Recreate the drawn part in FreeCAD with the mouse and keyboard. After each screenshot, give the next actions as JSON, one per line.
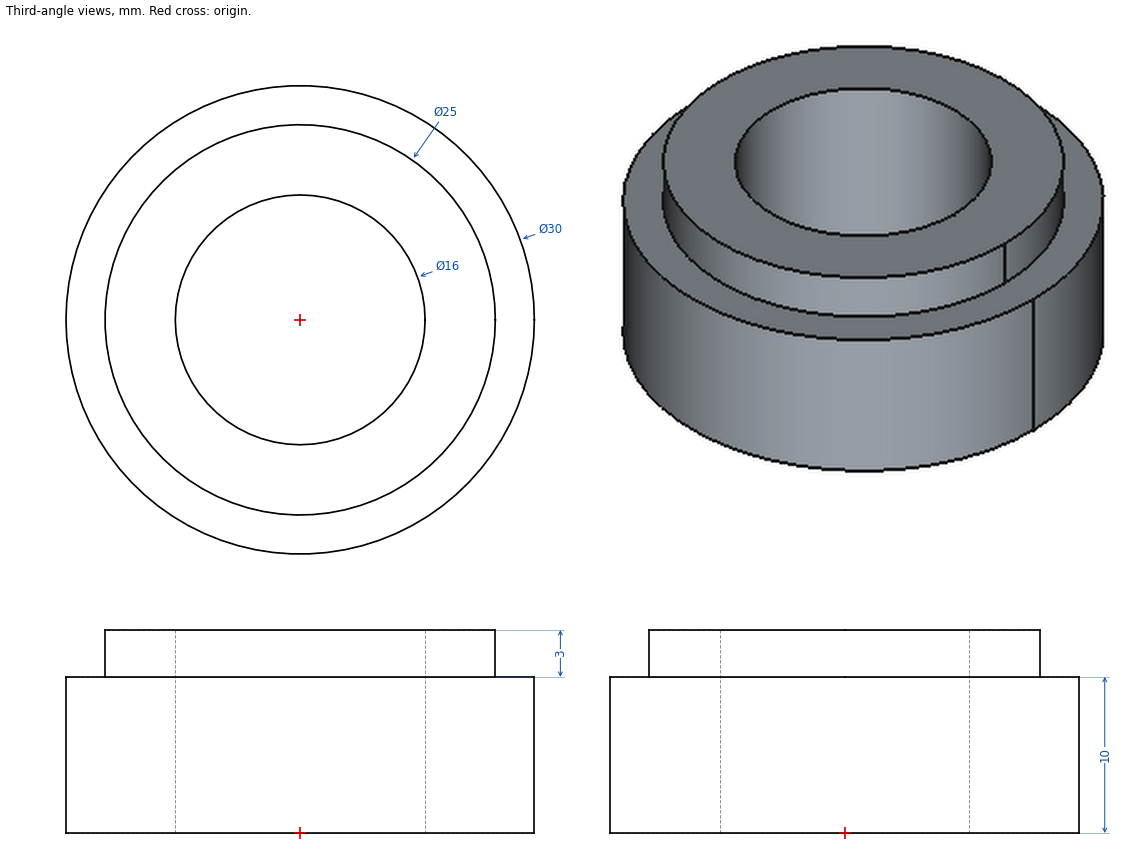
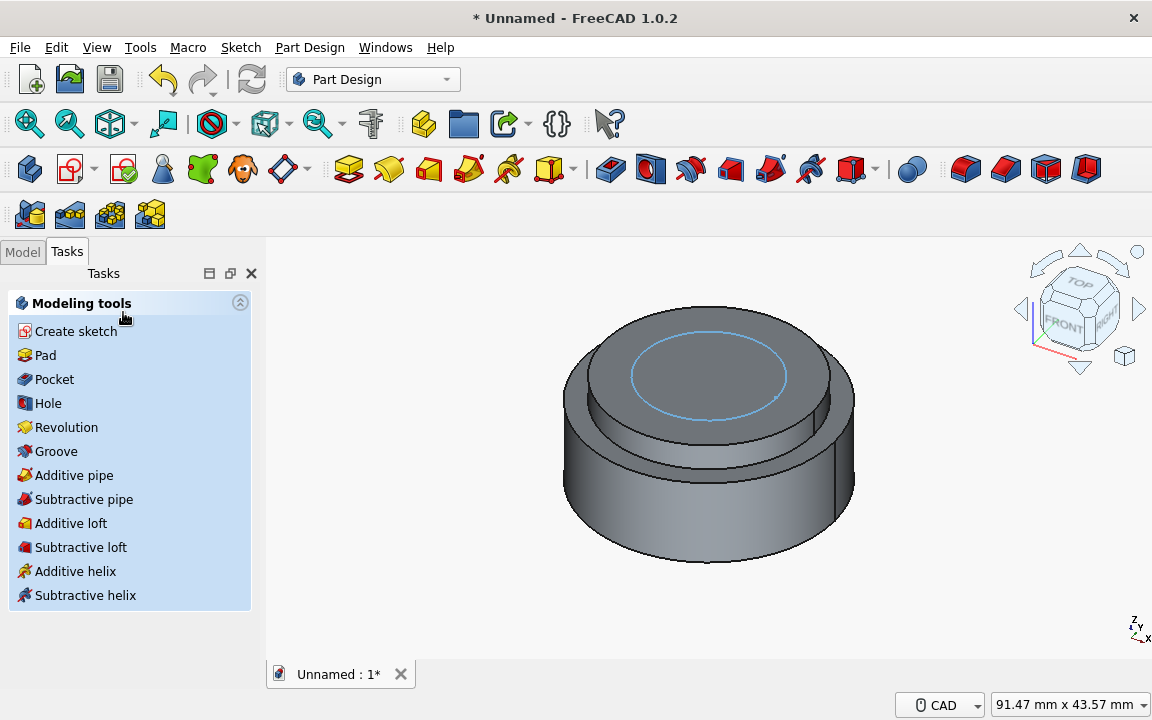
{"action": "left_click", "coordinate": [612, 170]}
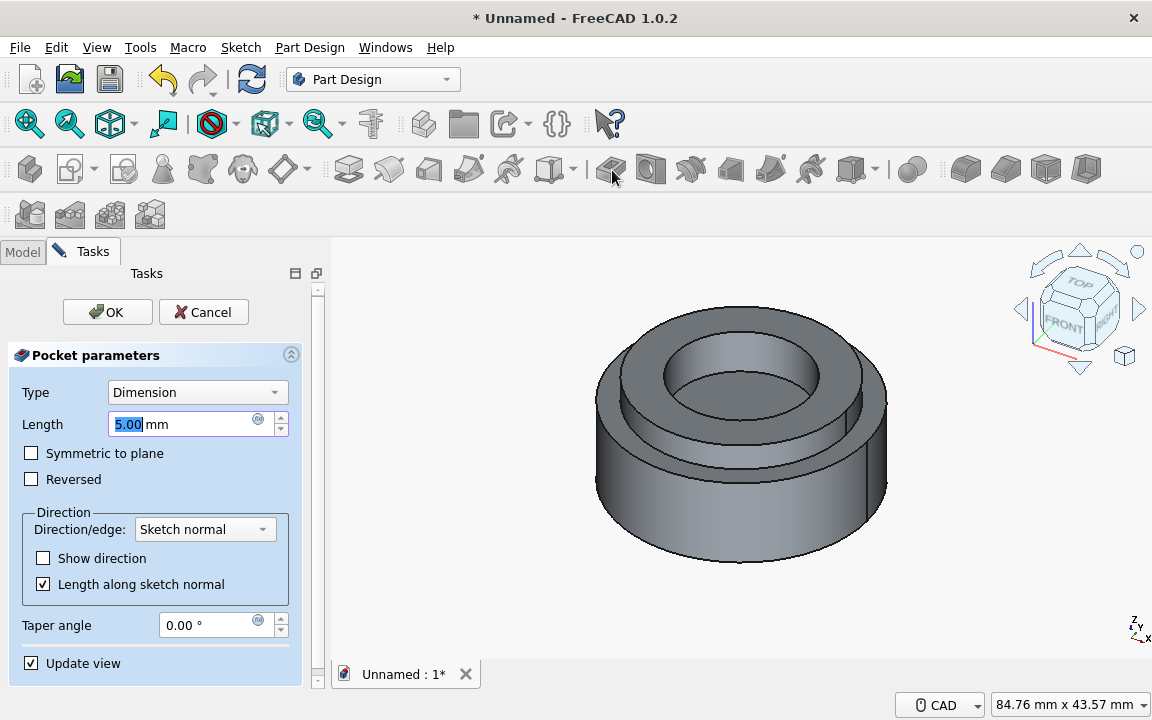
{"action": "left_click", "coordinate": [198, 392]}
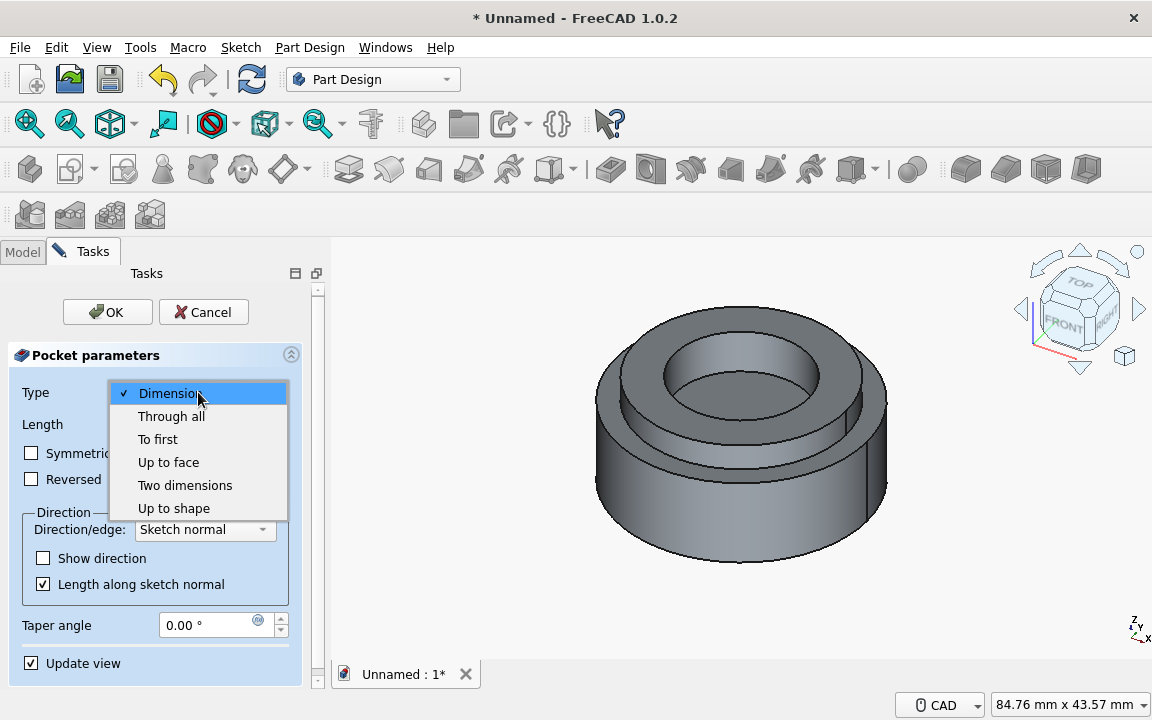
{"action": "left_click", "coordinate": [198, 416]}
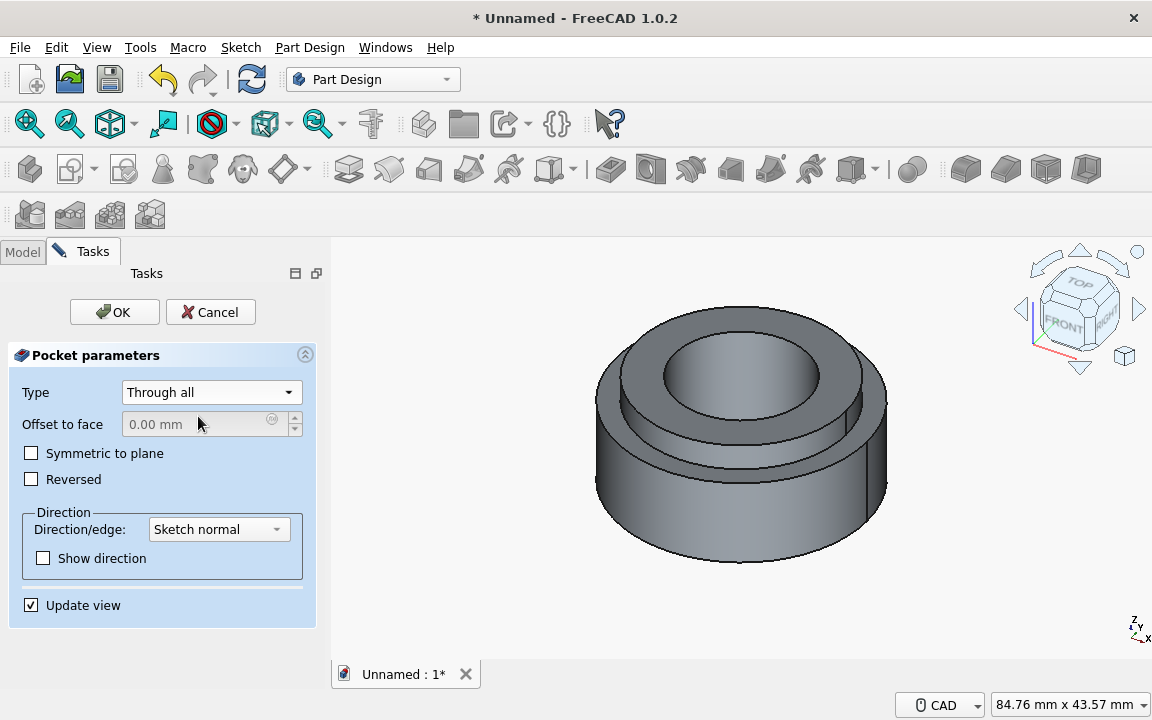
{"action": "left_click", "coordinate": [115, 312]}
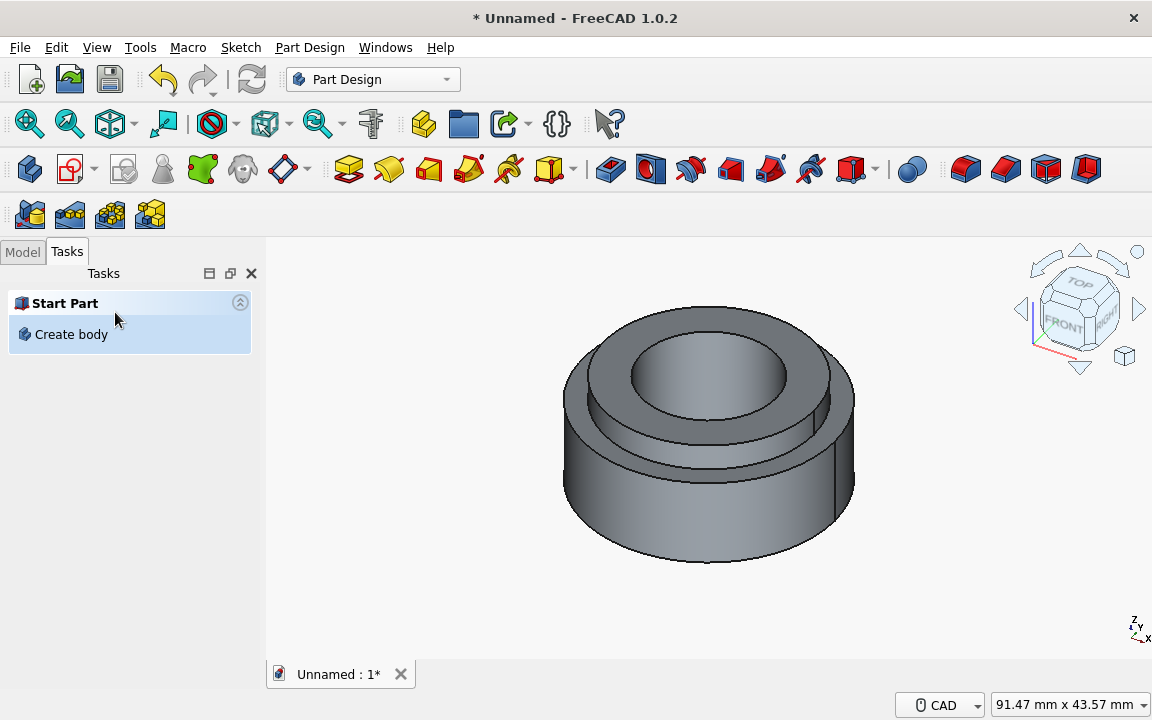
{"action": "key", "text": "0"}